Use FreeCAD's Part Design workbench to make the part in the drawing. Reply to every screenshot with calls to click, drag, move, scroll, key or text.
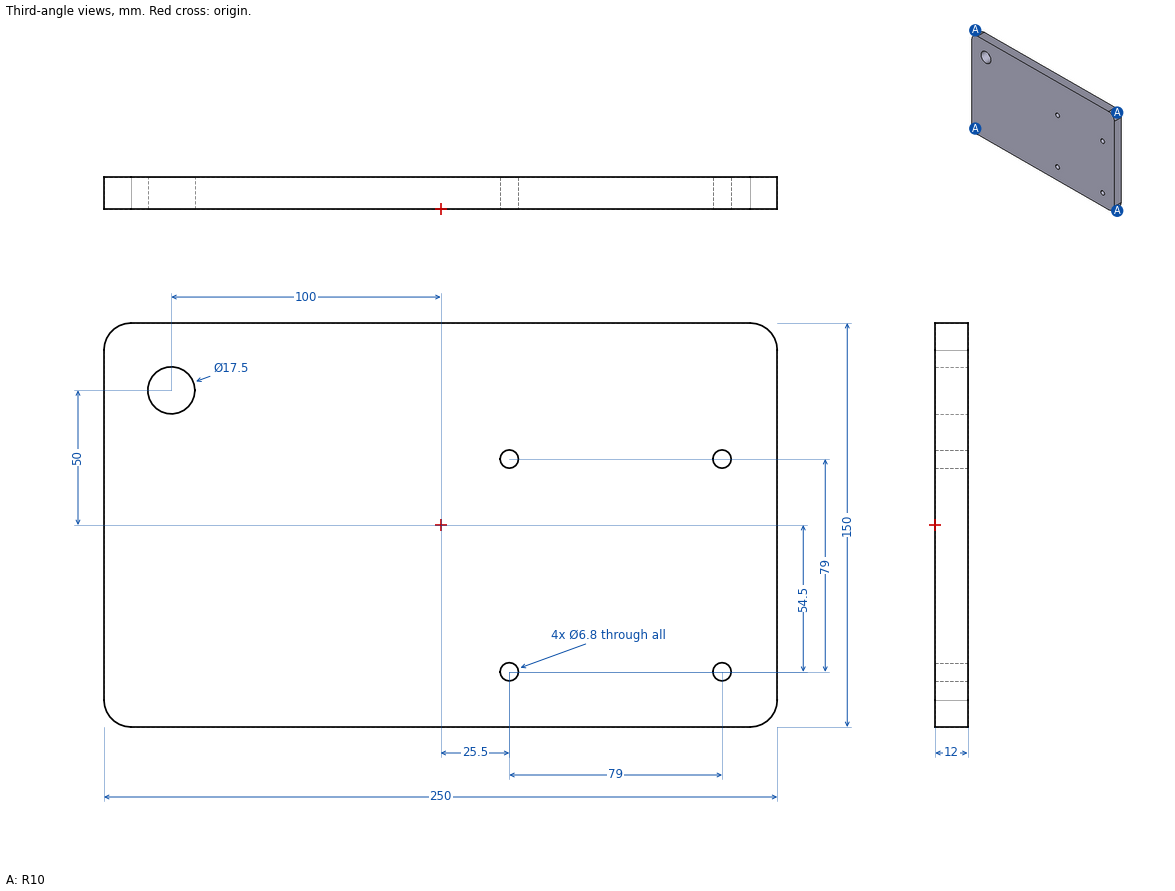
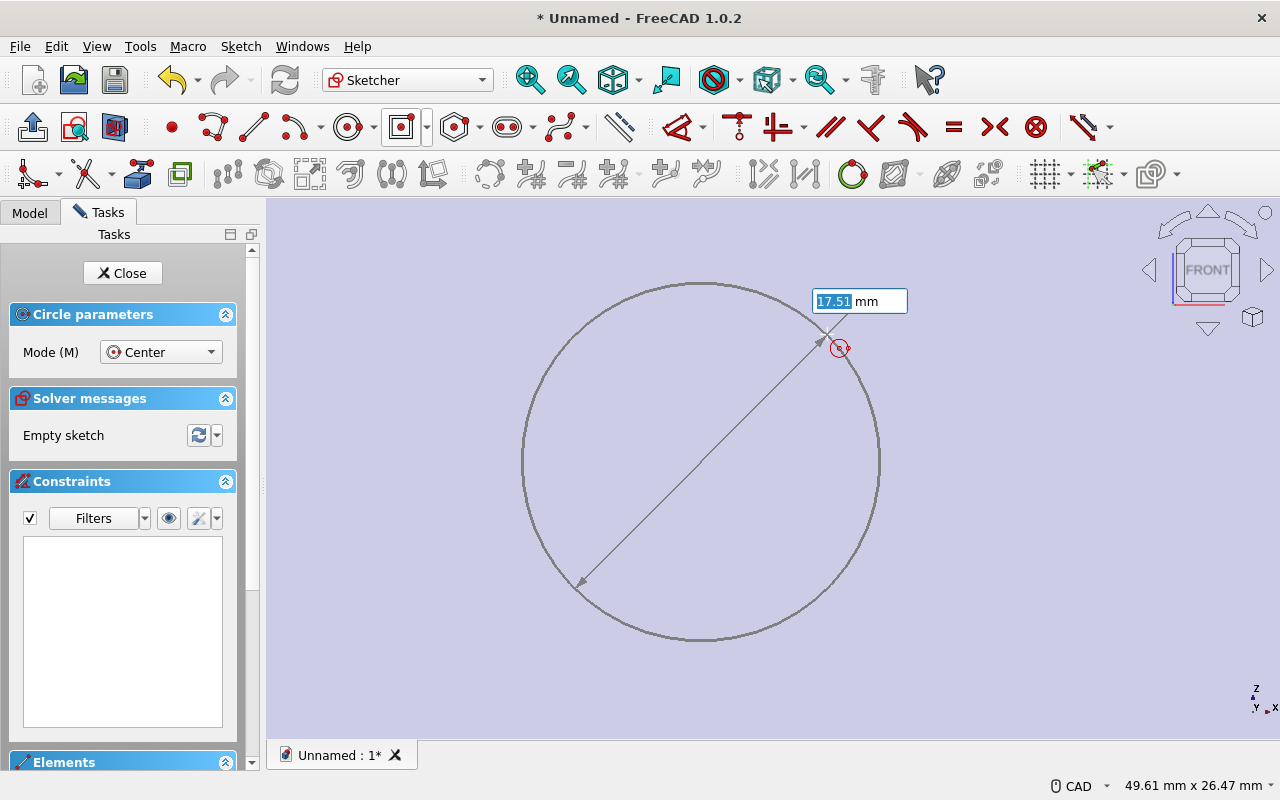
text(17.5)
key(Return)
key(Escape)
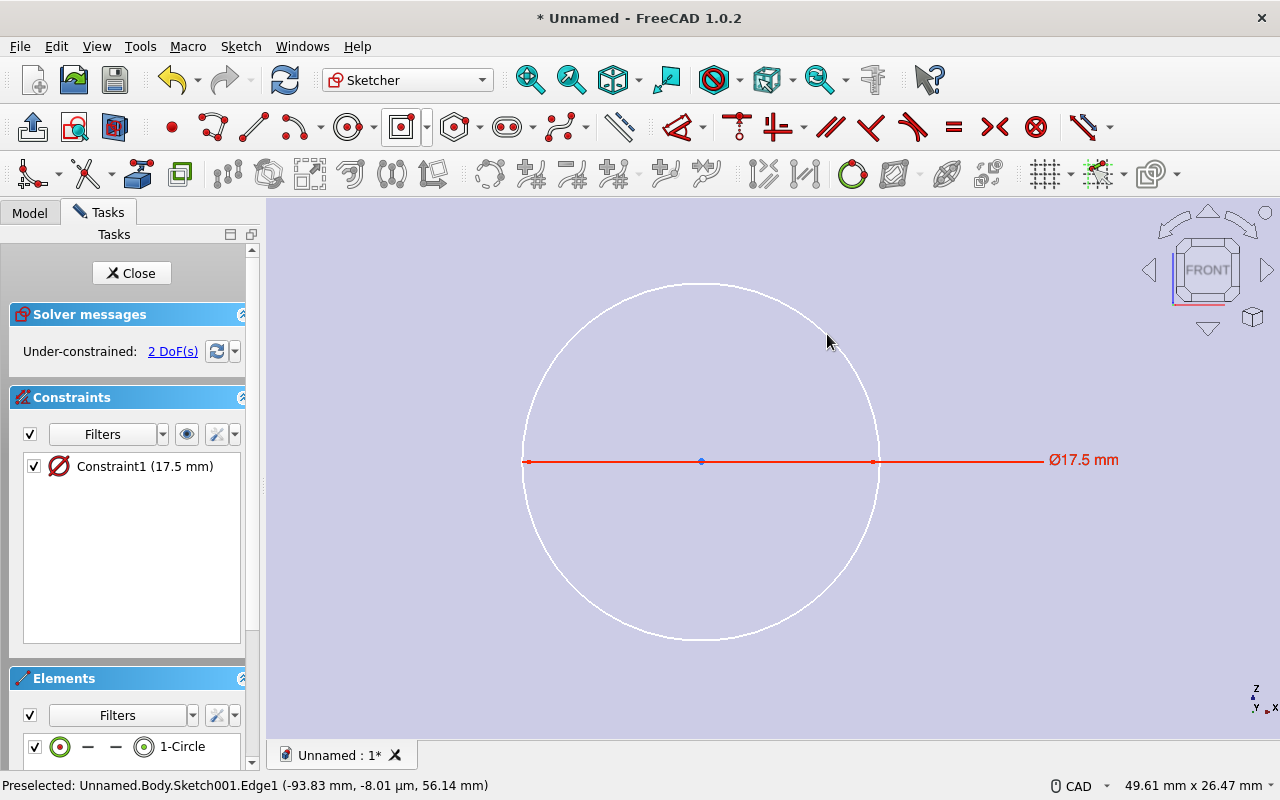
click(676, 128)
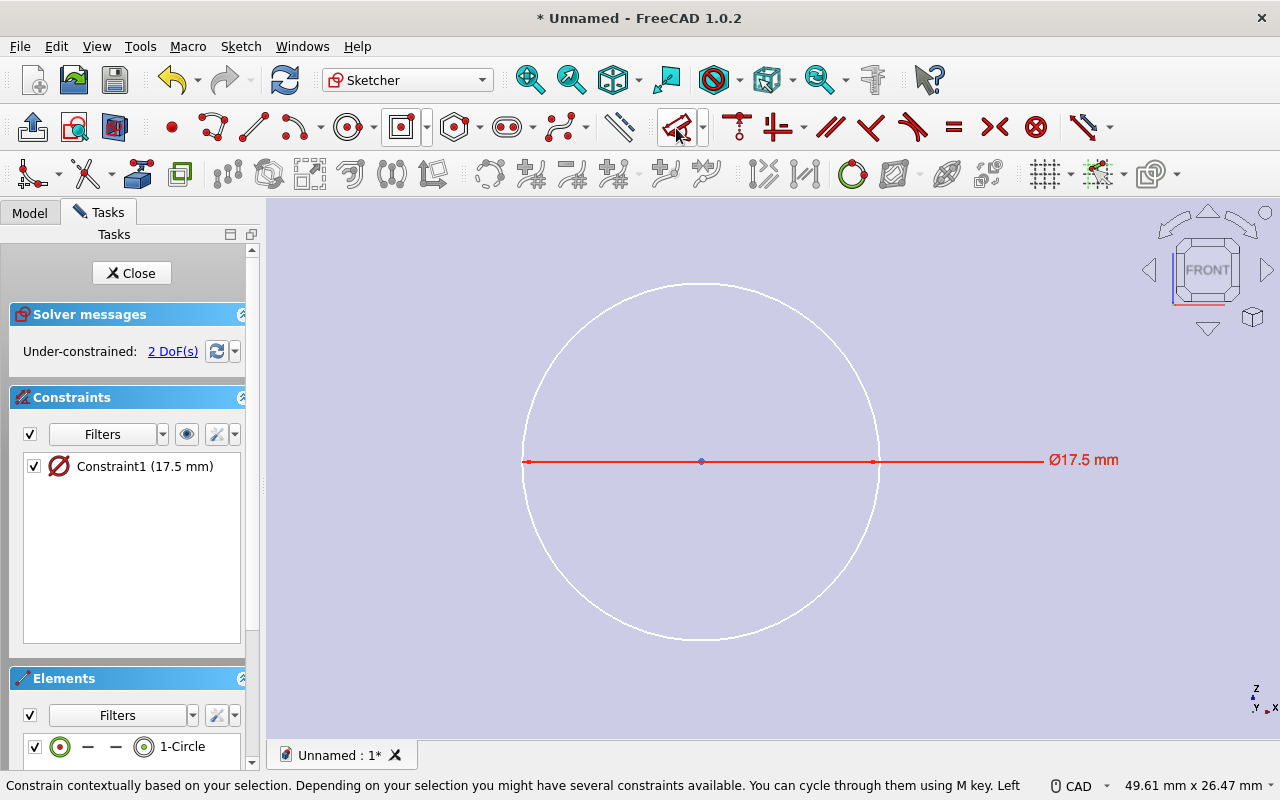
click(701, 462)
click(667, 587)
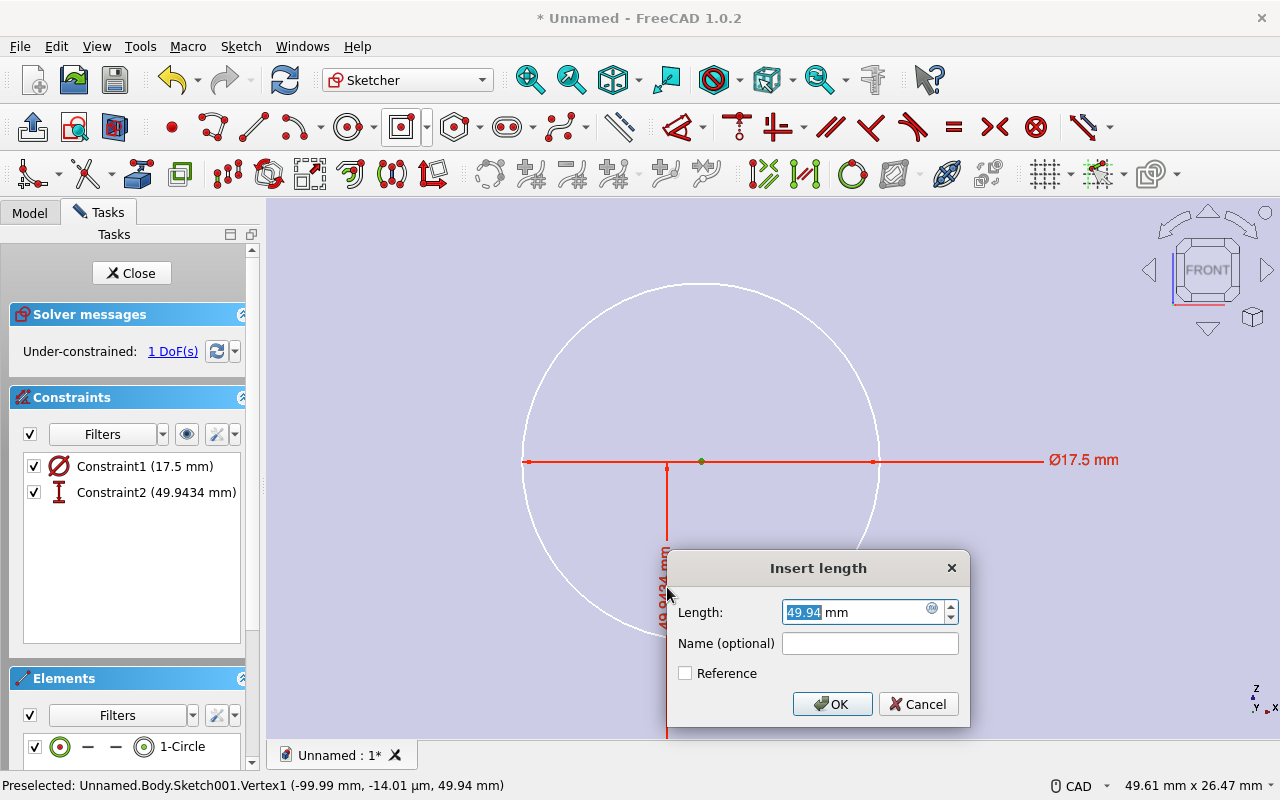
text(50)
key(Return)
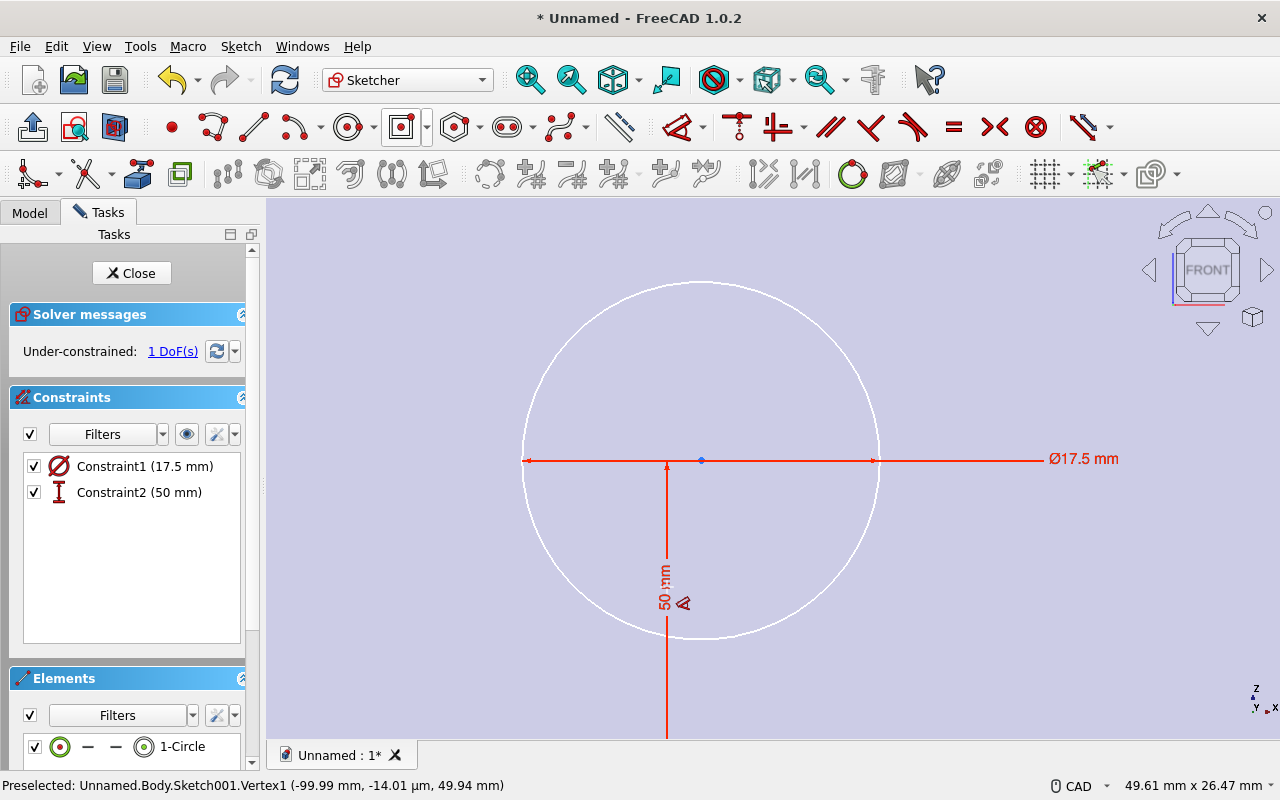
click(701, 461)
click(908, 427)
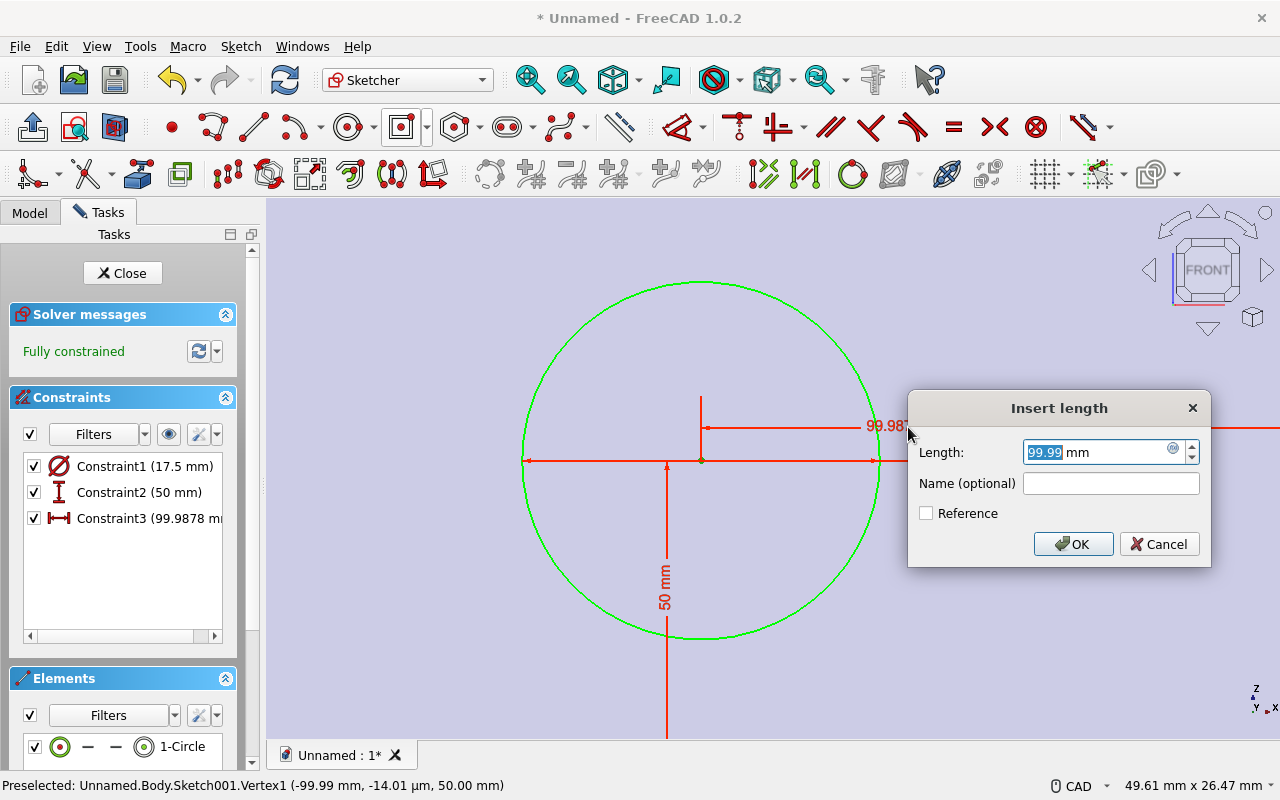
text(100)
key(Return)
key(Escape)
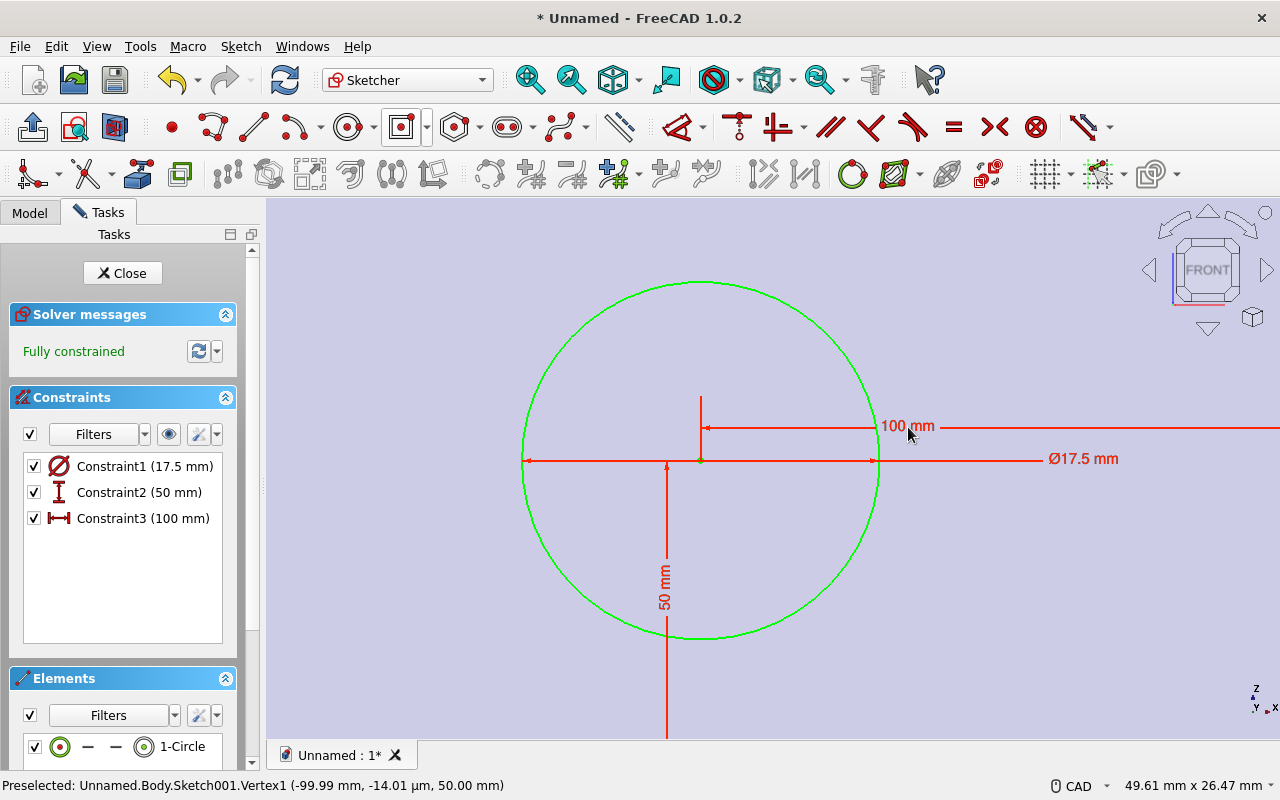
click(123, 273)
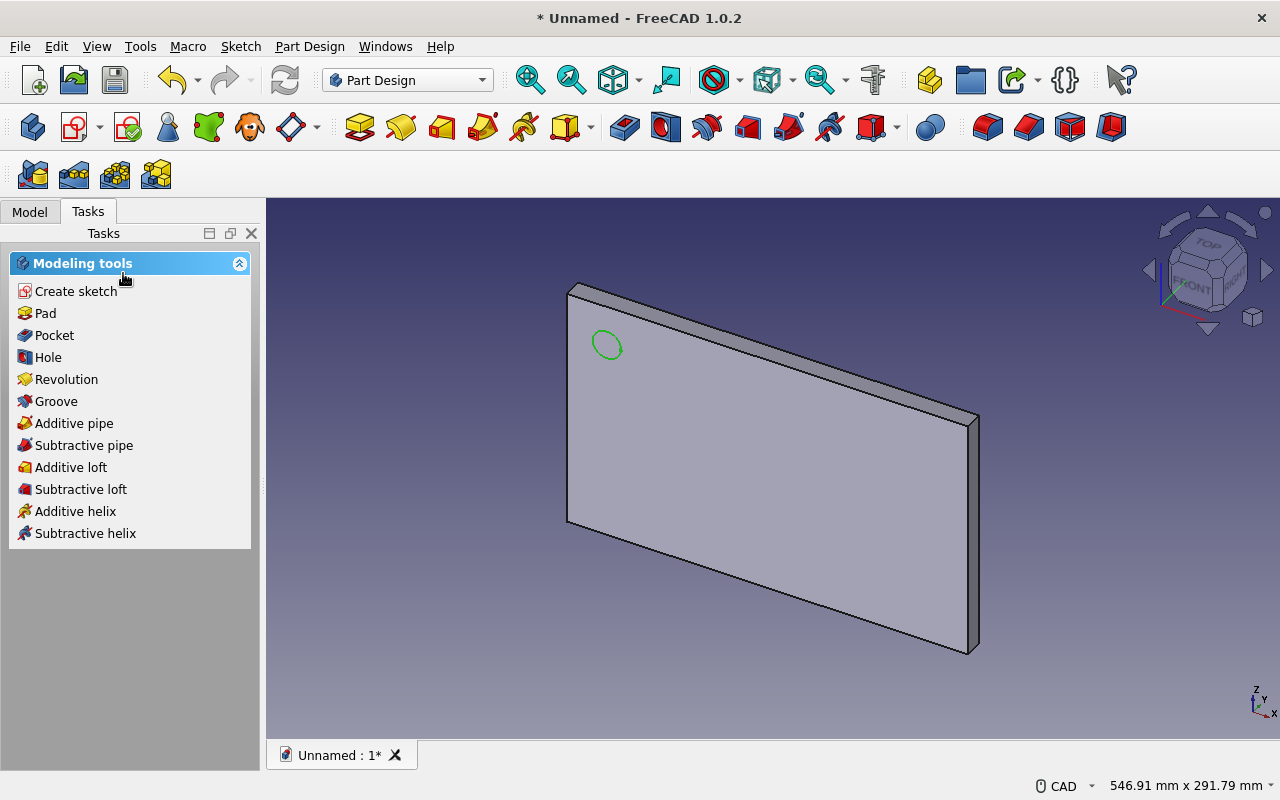
click(625, 128)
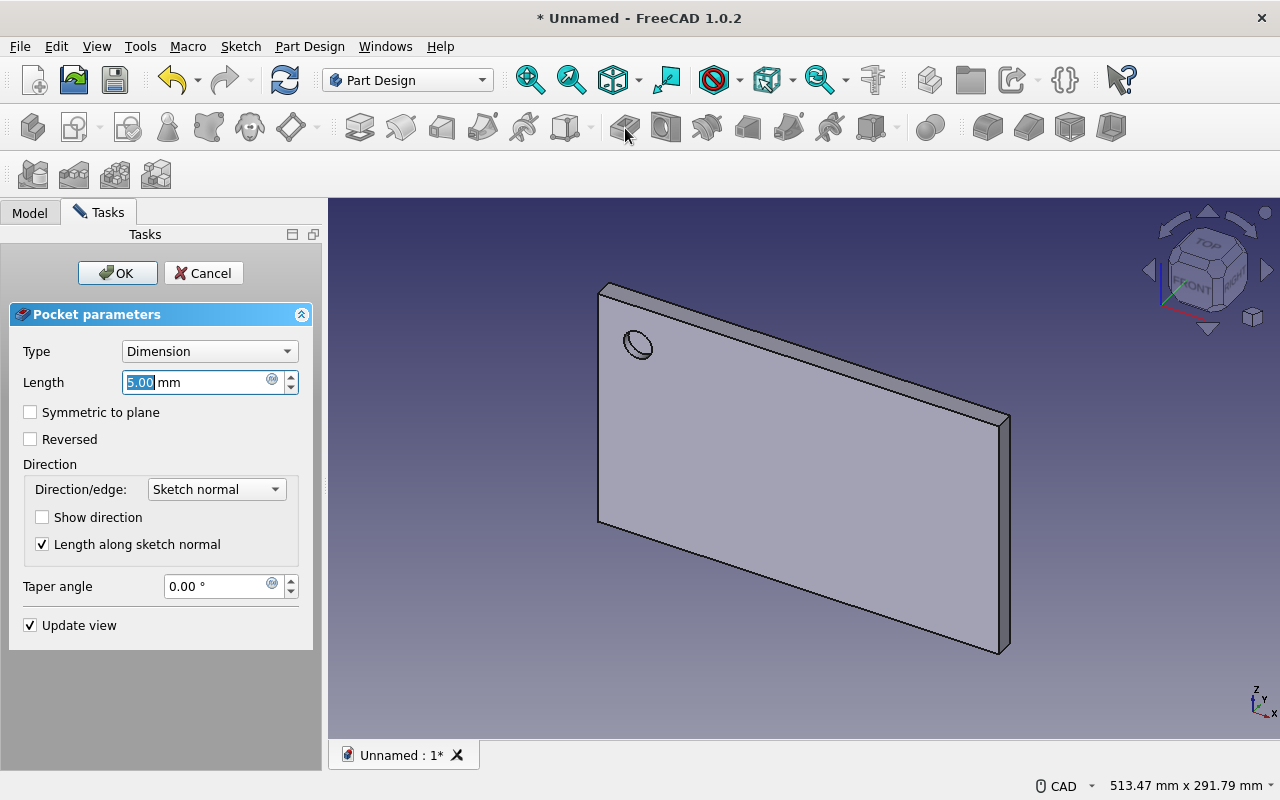
click(210, 352)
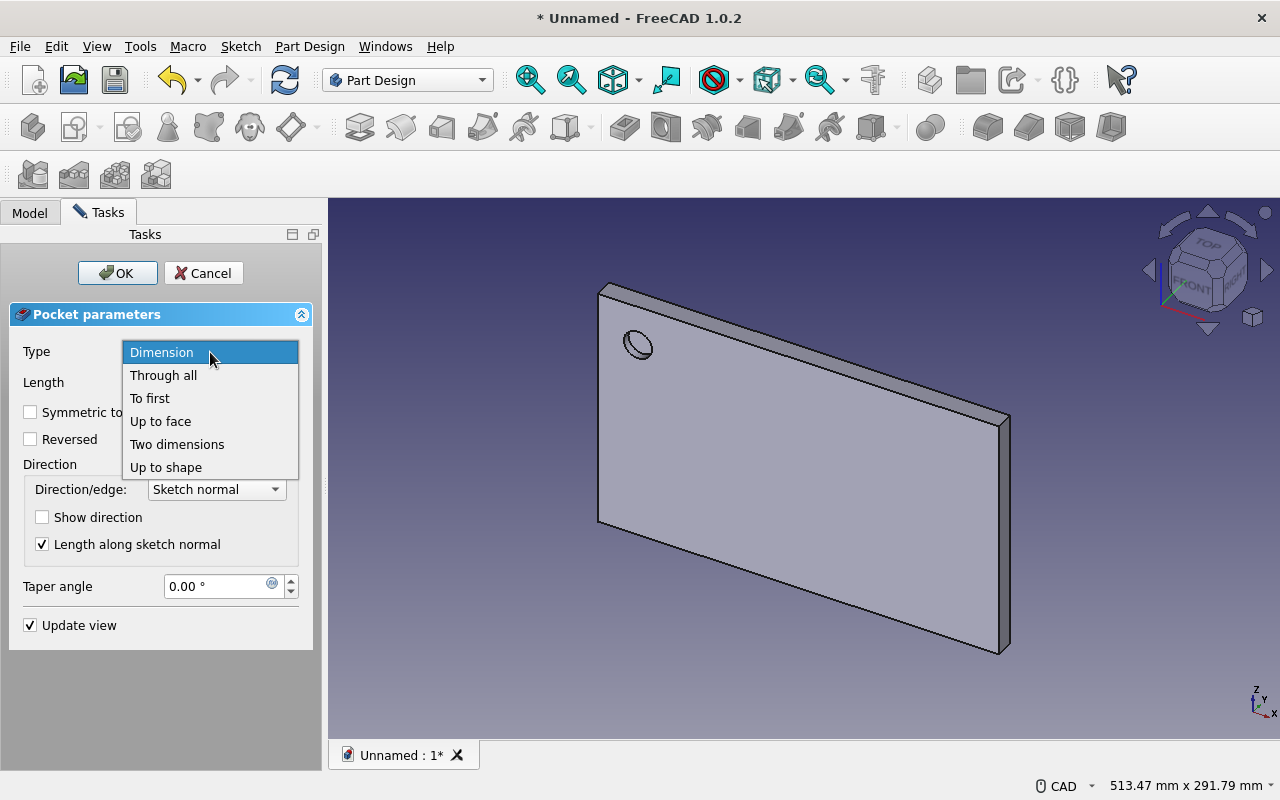
click(208, 376)